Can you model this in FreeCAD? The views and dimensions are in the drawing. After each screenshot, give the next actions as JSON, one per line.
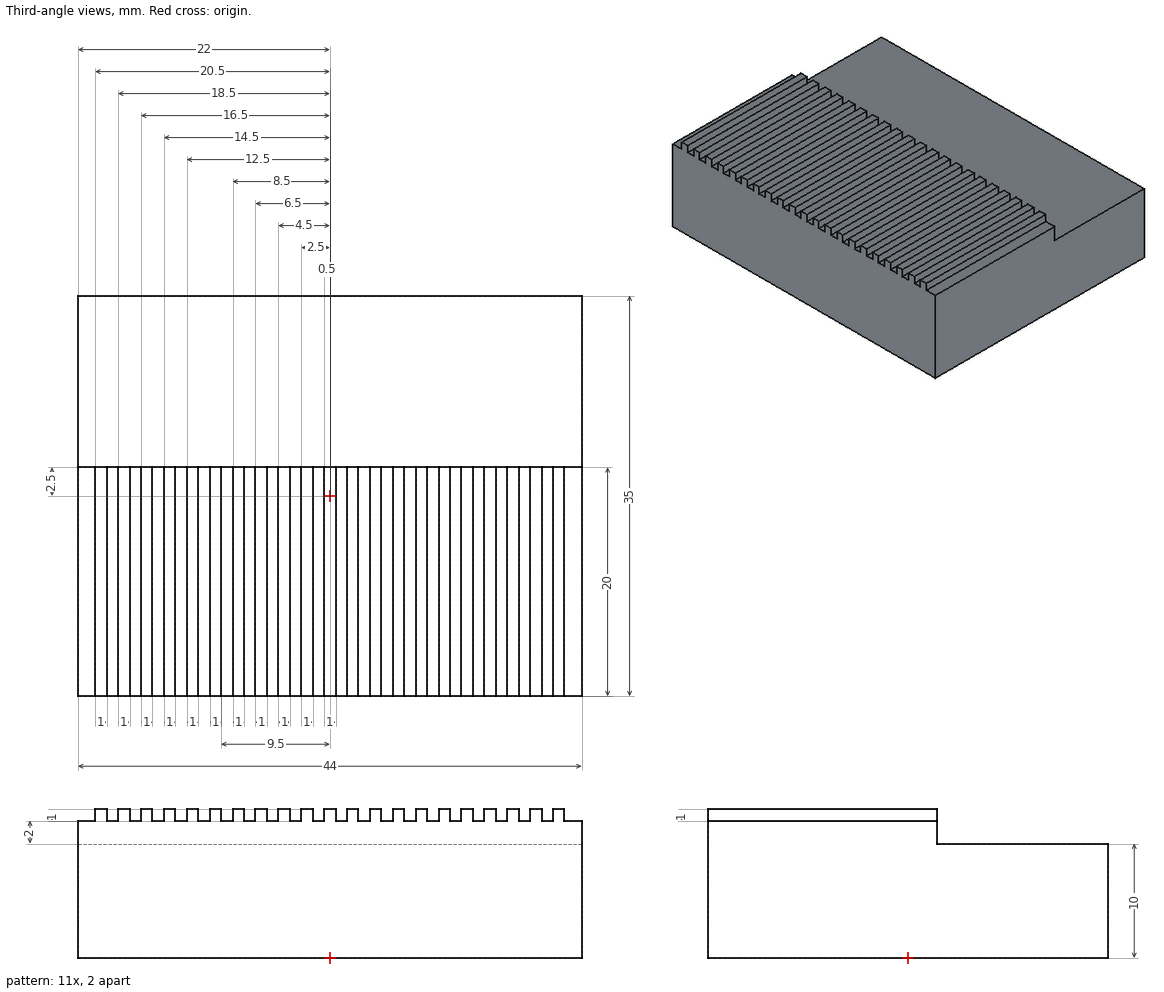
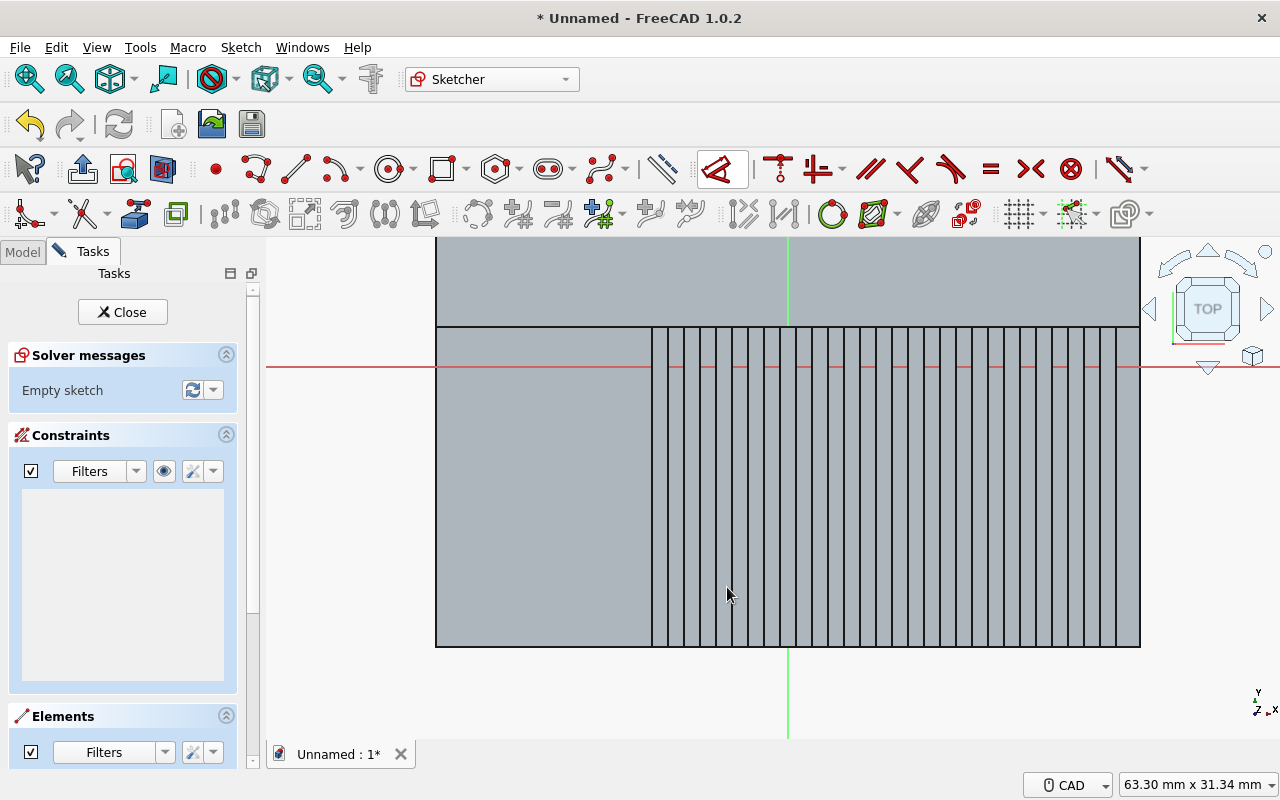
{"action": "left_click", "coordinate": [442, 170]}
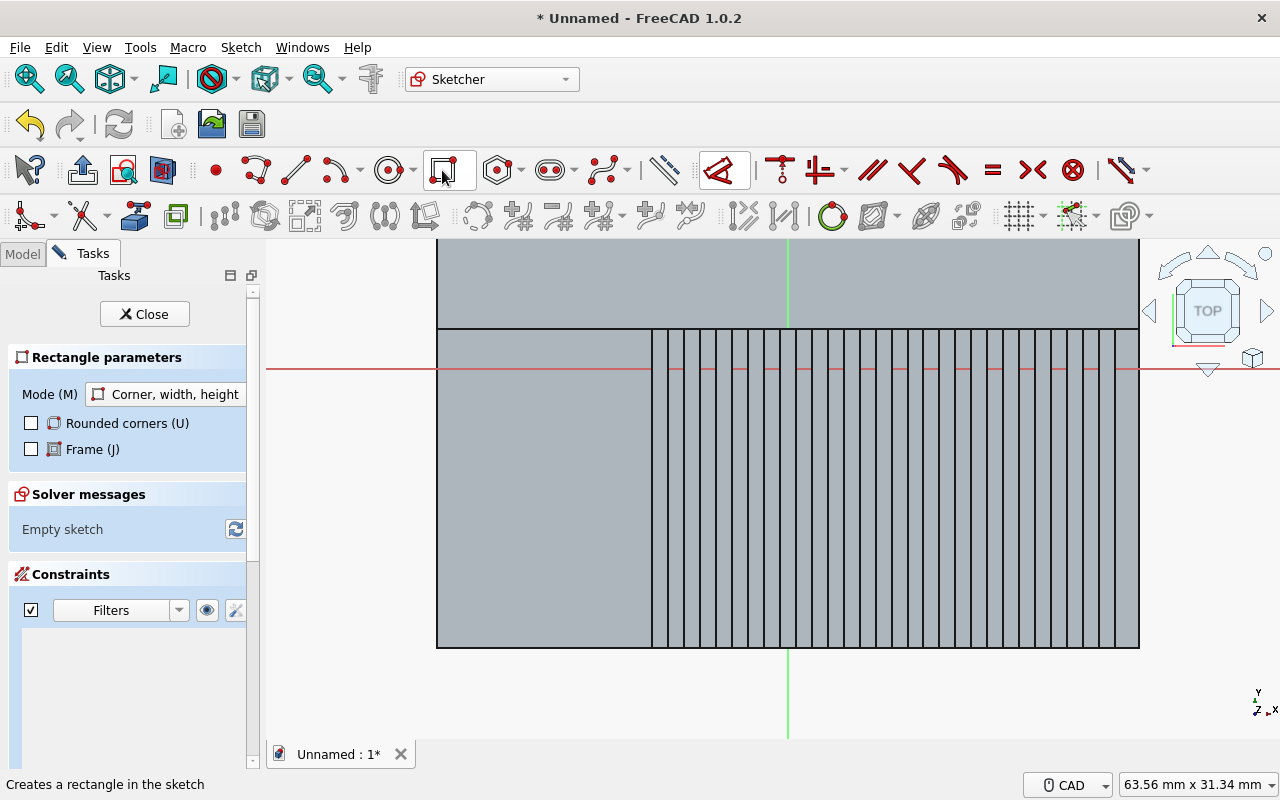
{"action": "left_click", "coordinate": [620, 329]}
{"action": "mouse_move", "coordinate": [636, 648]}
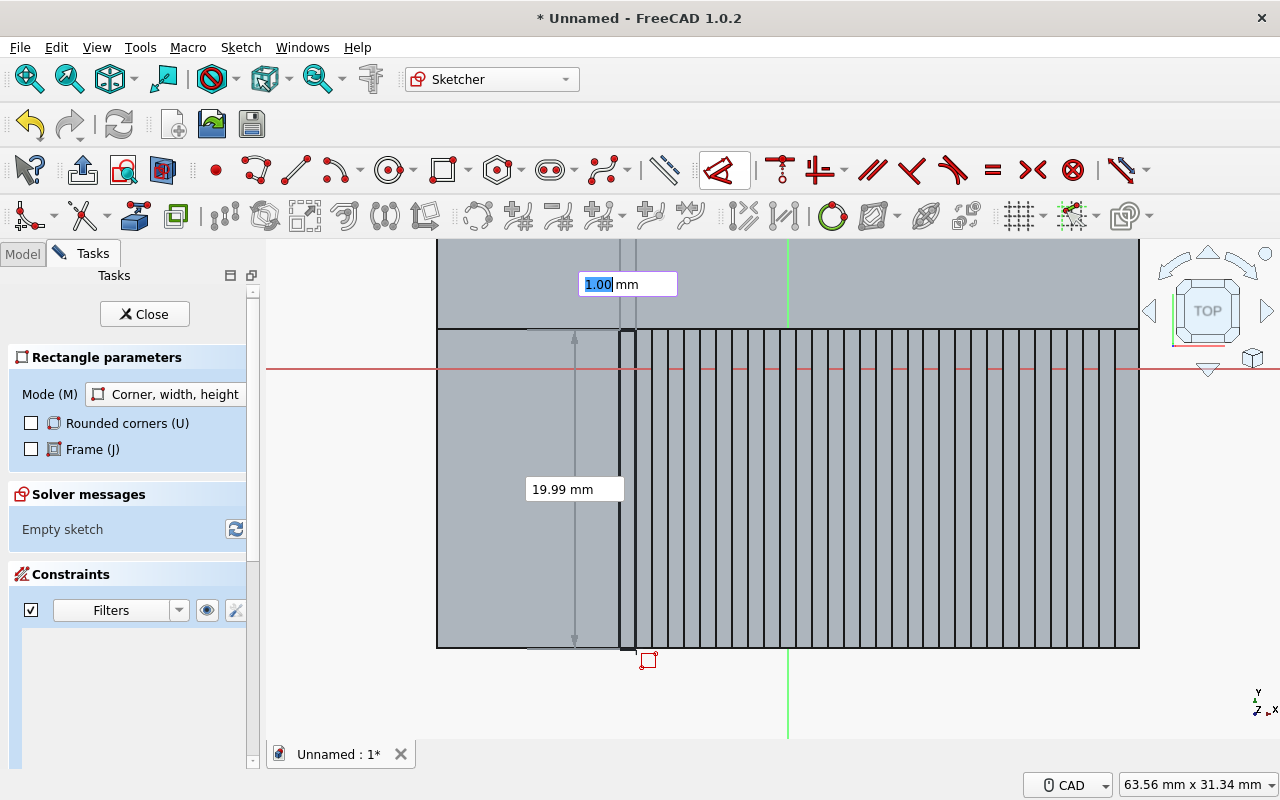
{"action": "type", "text": "1"}
{"action": "key", "text": "Tab"}
{"action": "type", "text": "20"}
{"action": "key", "text": "Return"}
{"action": "key", "text": "Escape"}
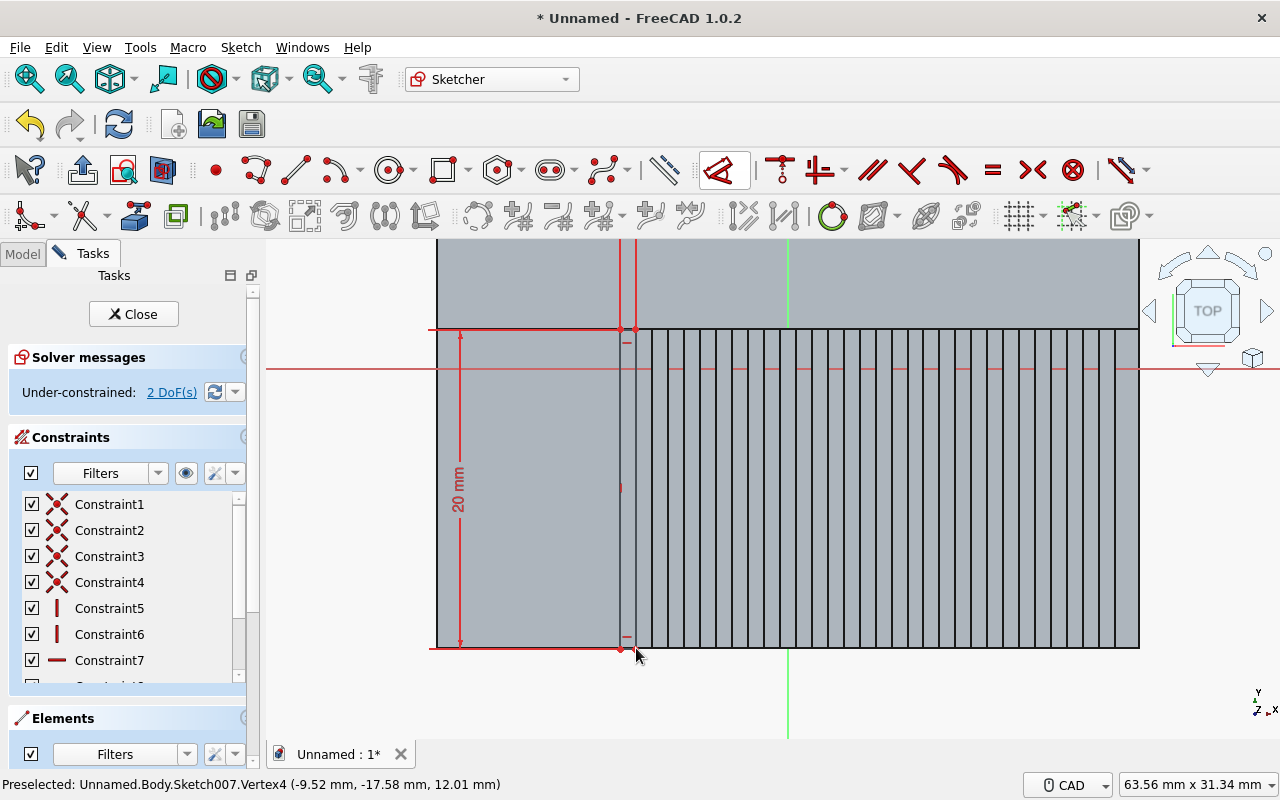
{"action": "left_click", "coordinate": [620, 330]}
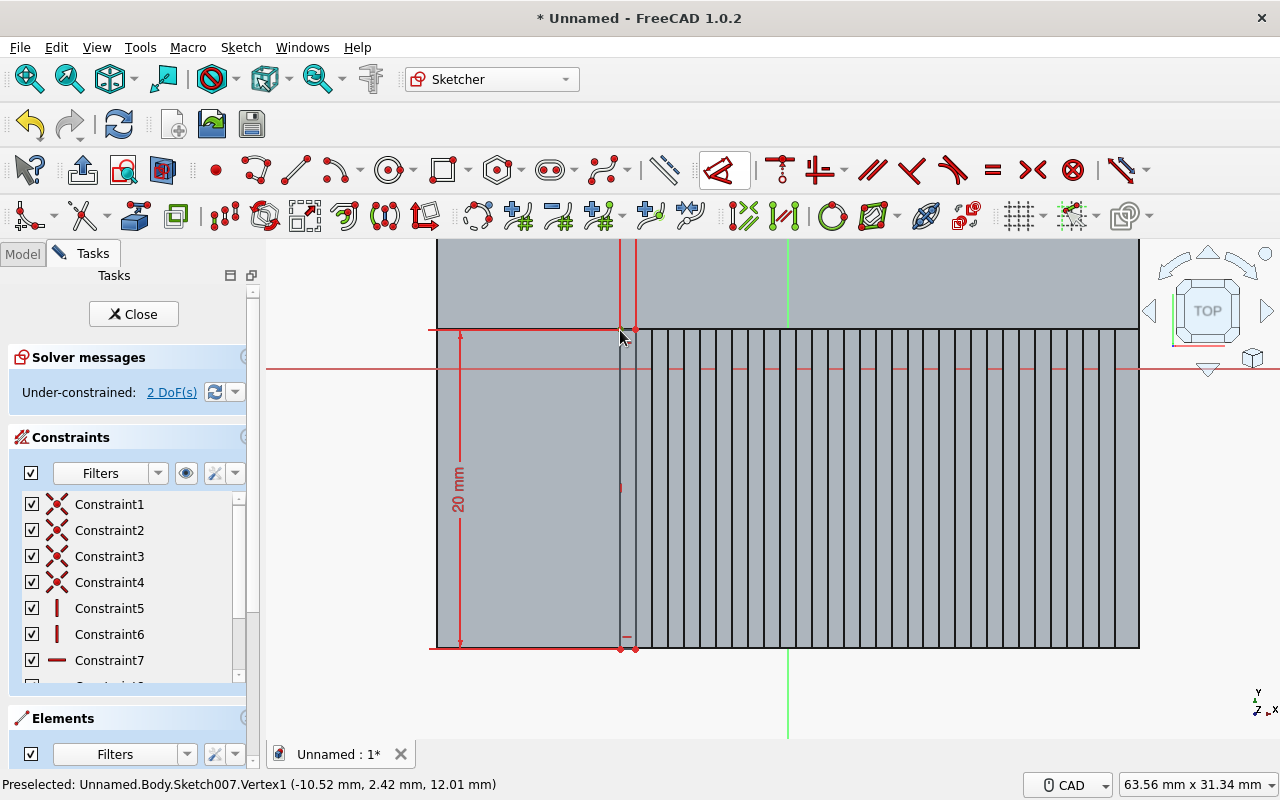
{"action": "left_click", "coordinate": [744, 170]}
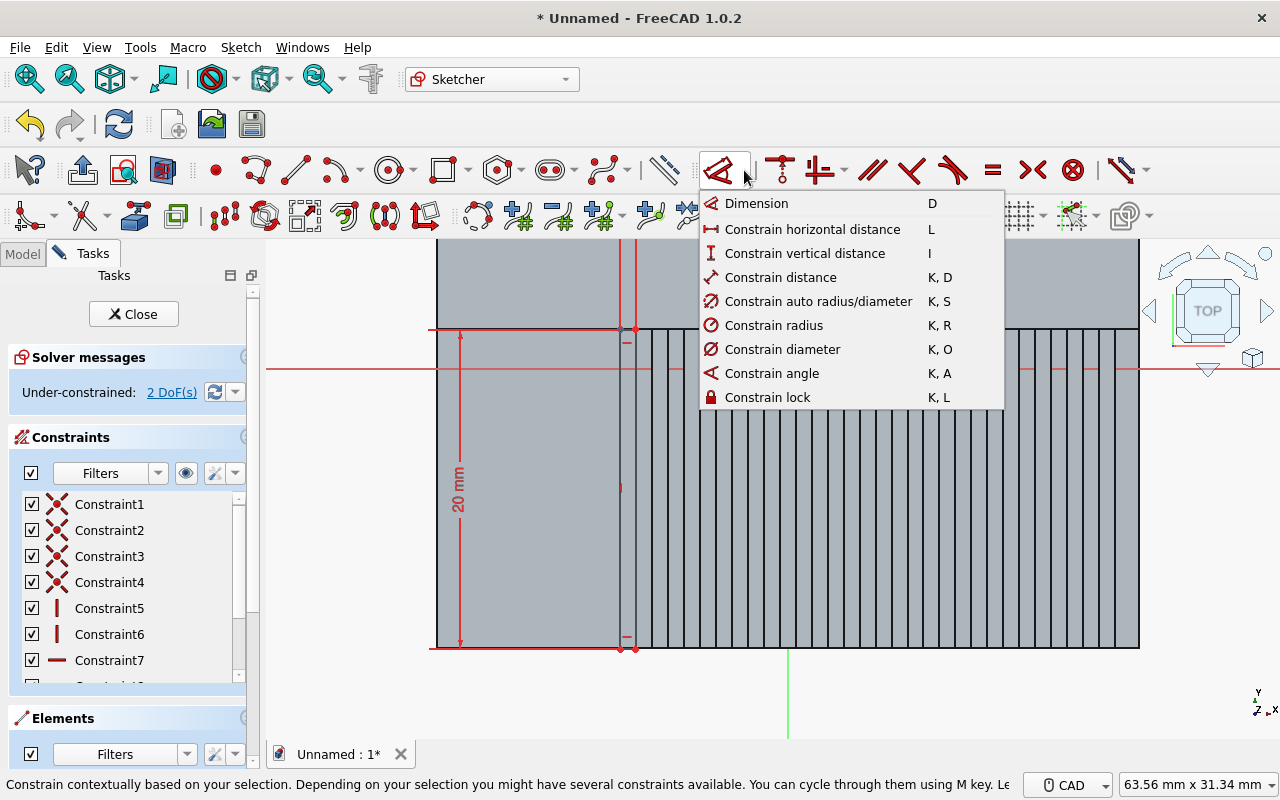
{"action": "left_click", "coordinate": [852, 253]}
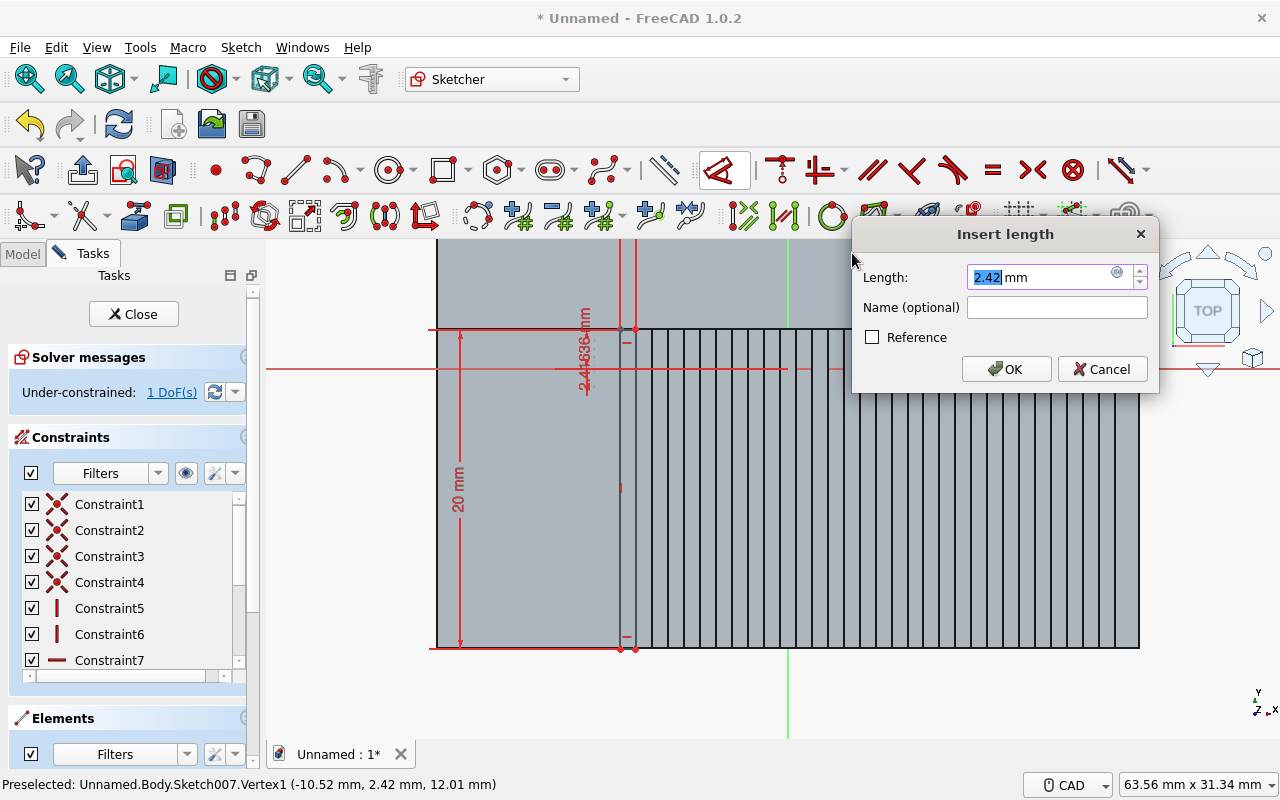
{"action": "type", "text": "2.5"}
{"action": "key", "text": "Return"}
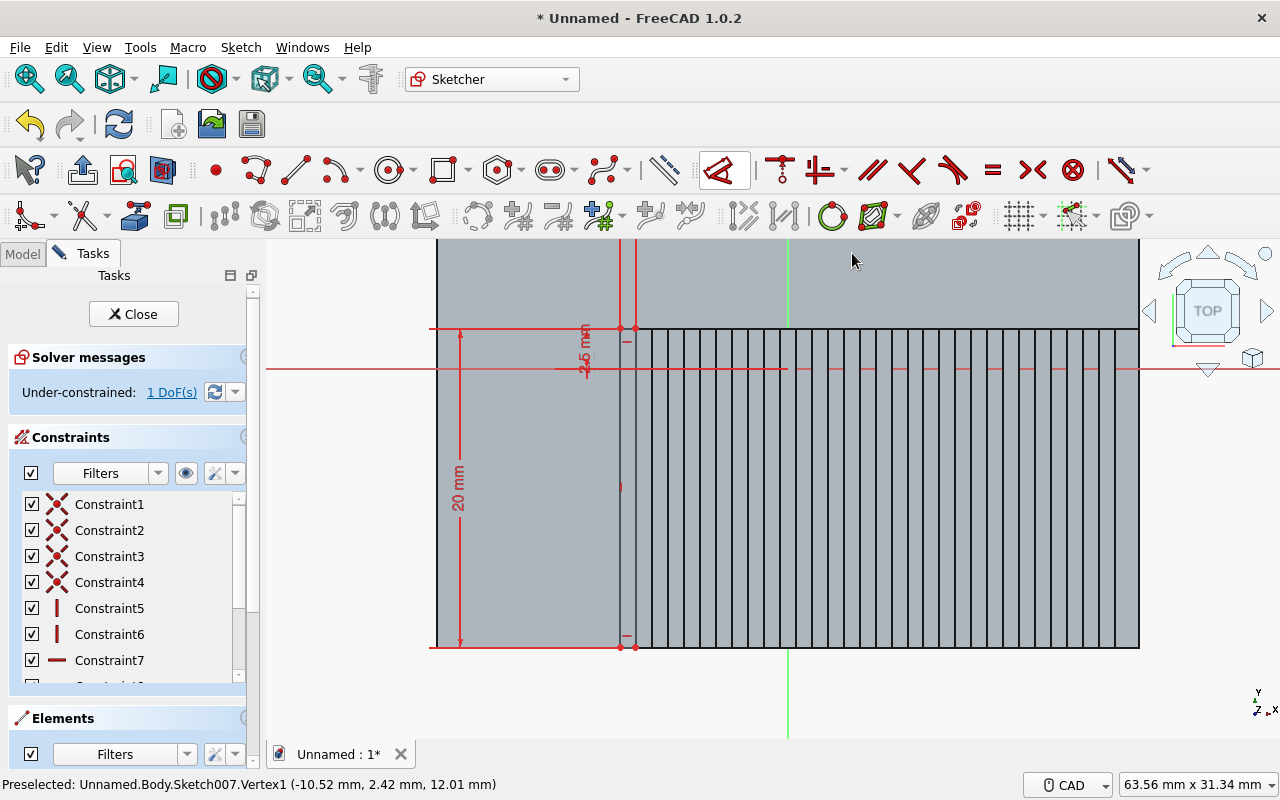
{"action": "left_click", "coordinate": [636, 648]}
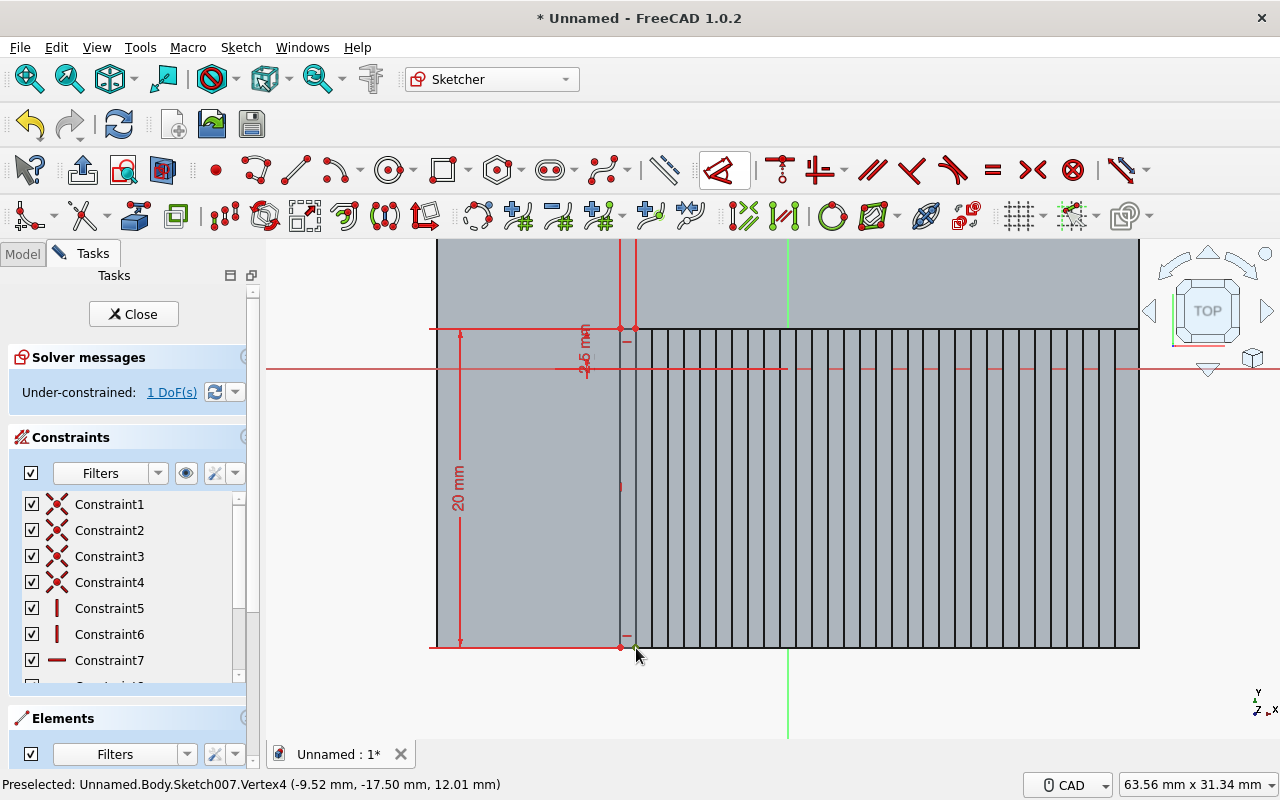
{"action": "left_click", "coordinate": [744, 170]}